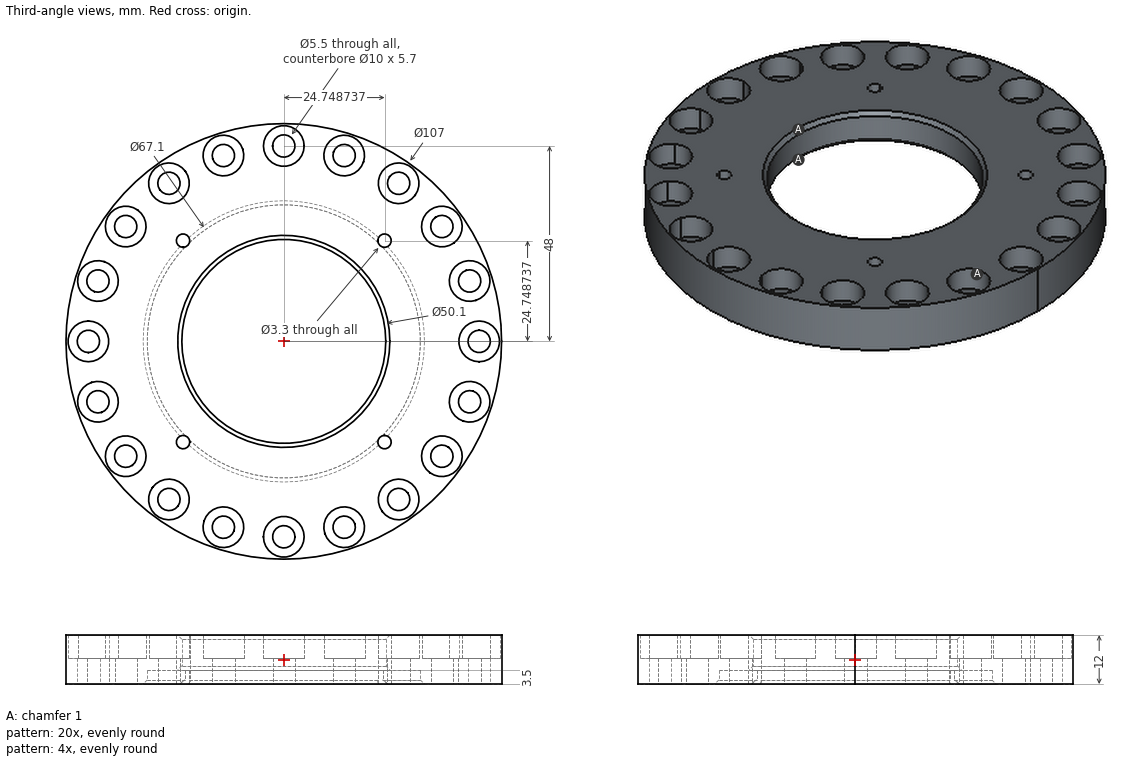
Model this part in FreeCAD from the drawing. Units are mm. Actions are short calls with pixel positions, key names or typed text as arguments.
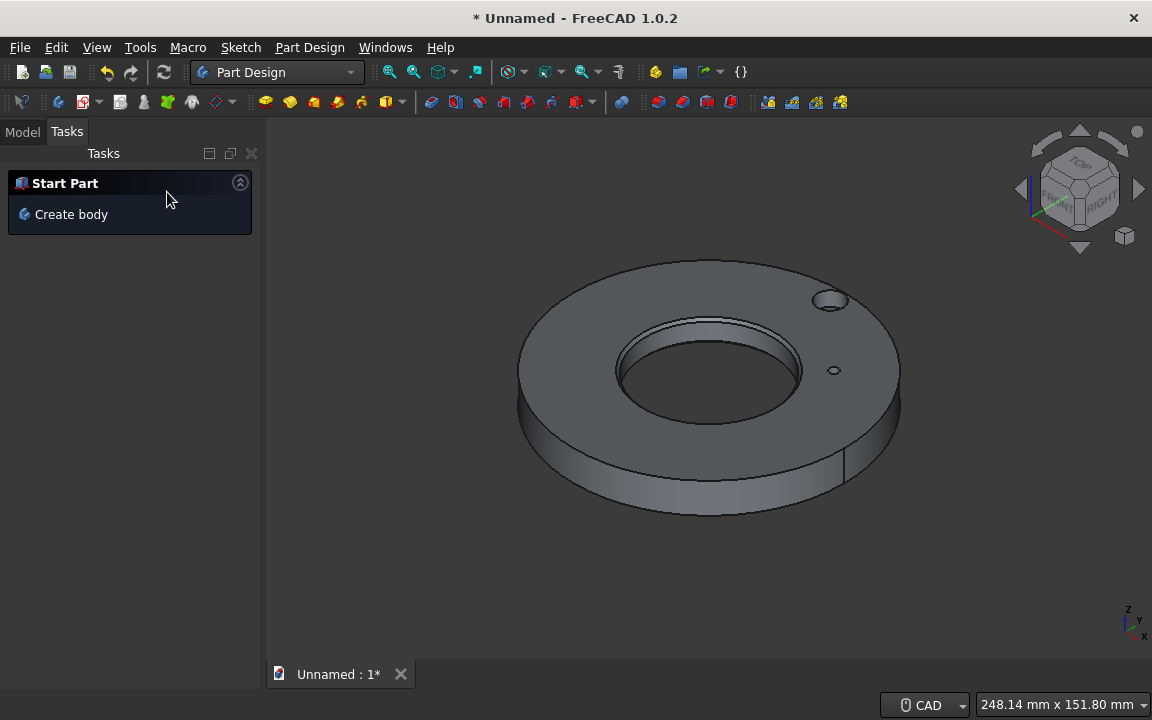
click(23, 131)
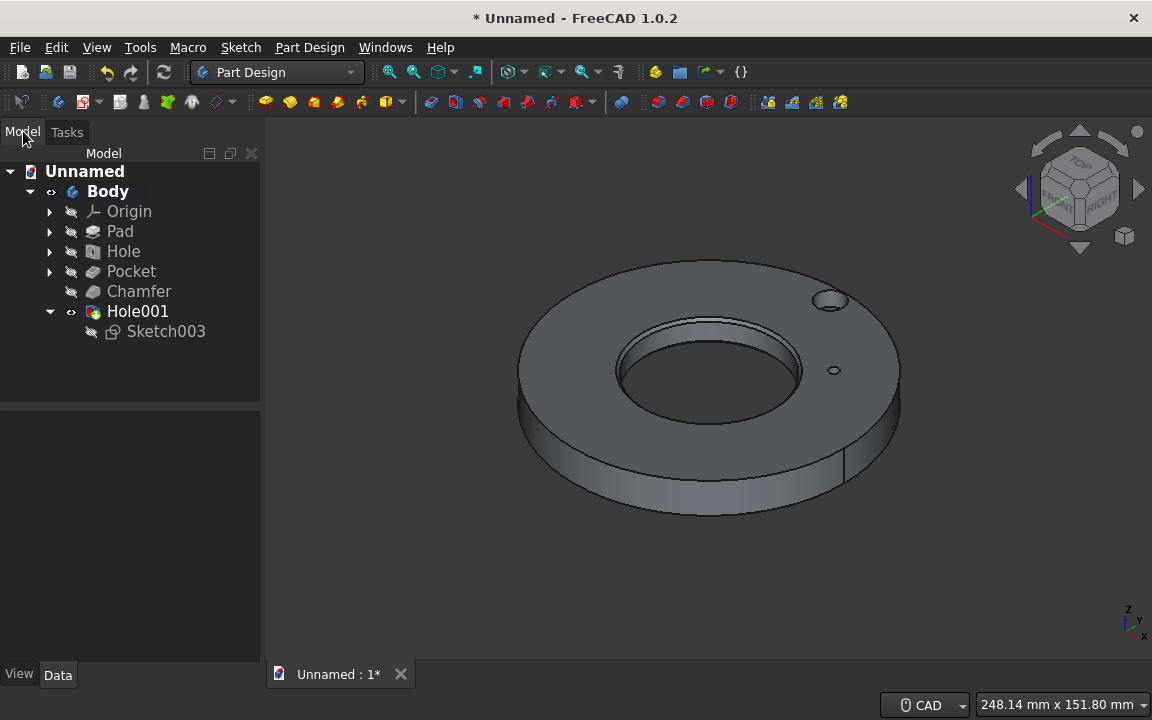
click(116, 252)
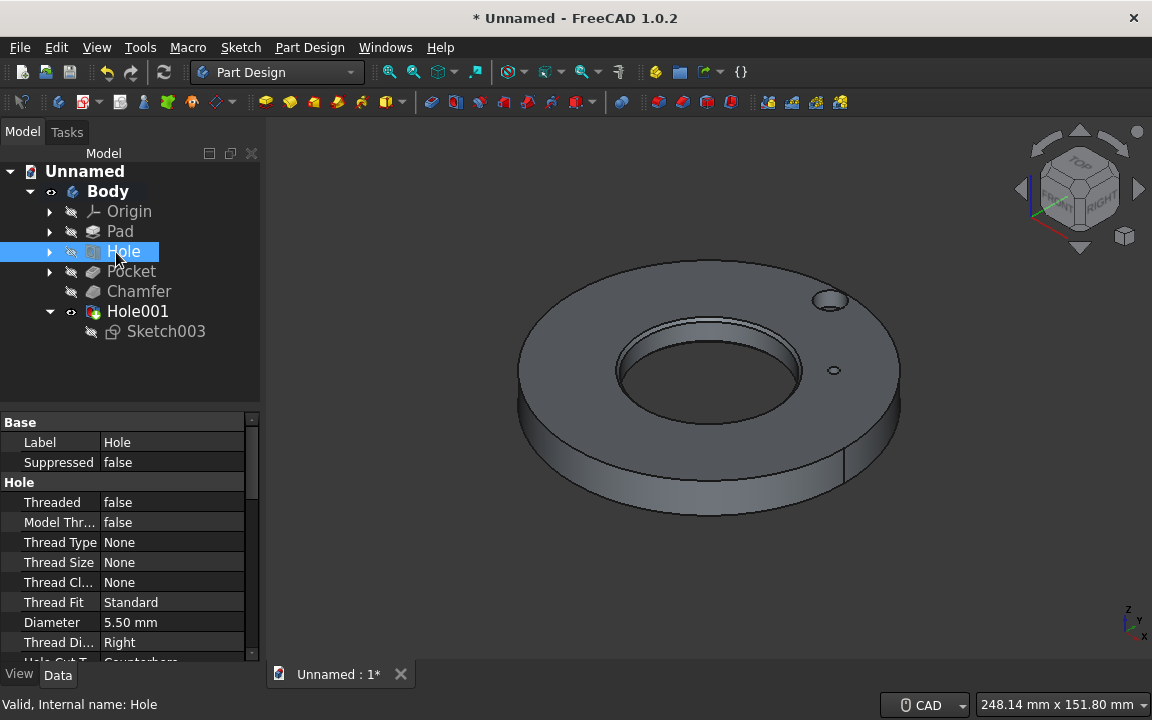
click(816, 102)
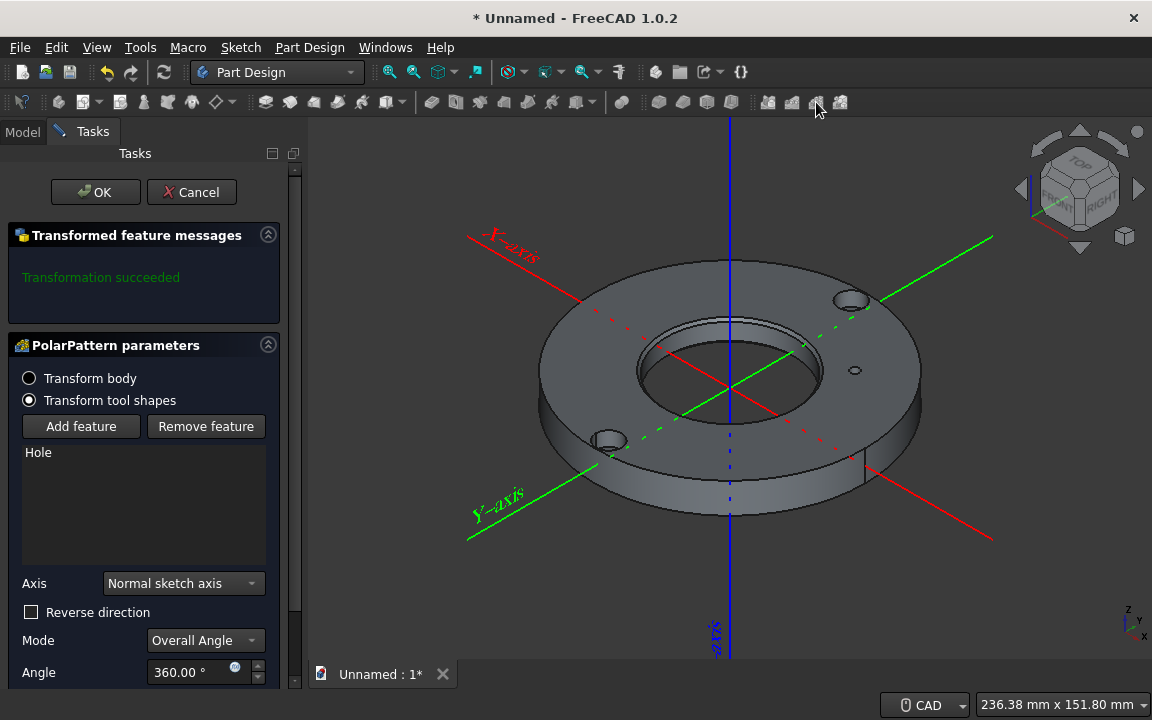
click(184, 584)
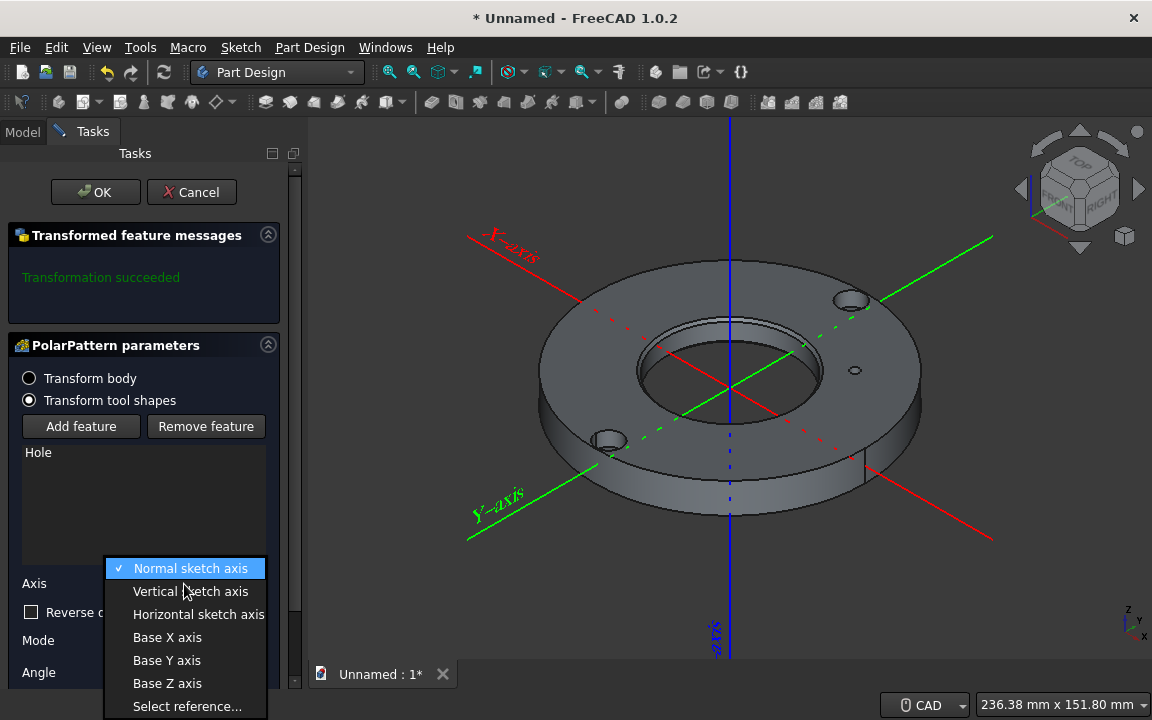
click(184, 684)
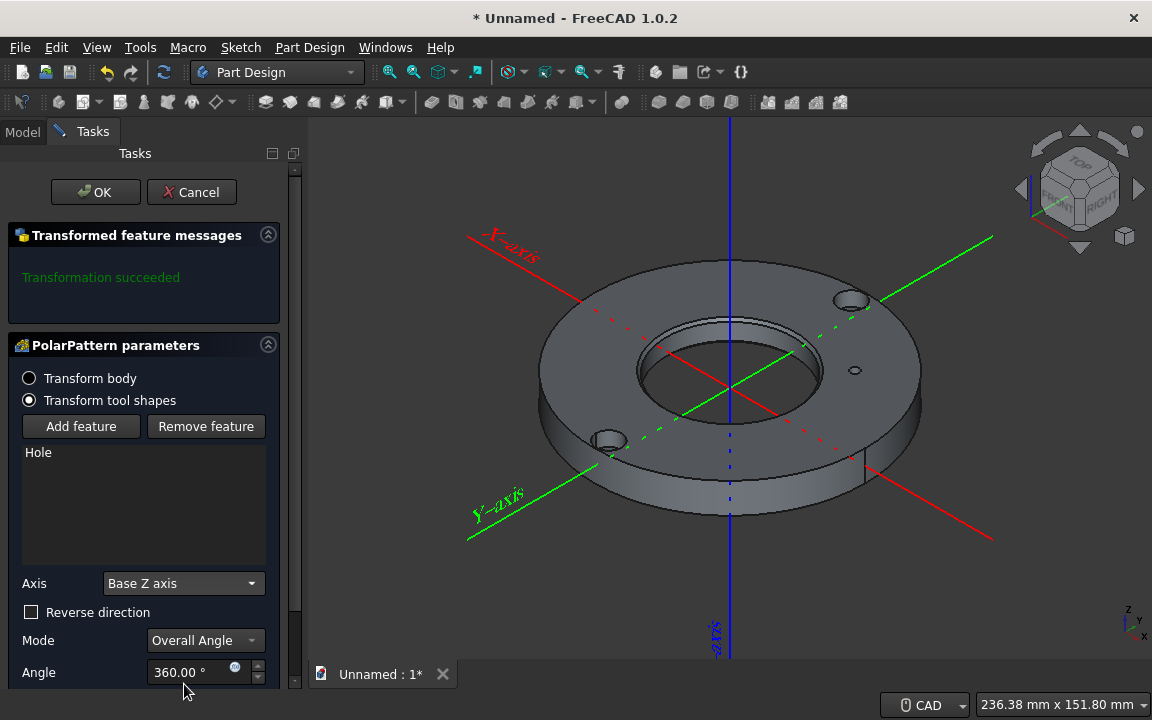
scroll(295, 426, down, 2)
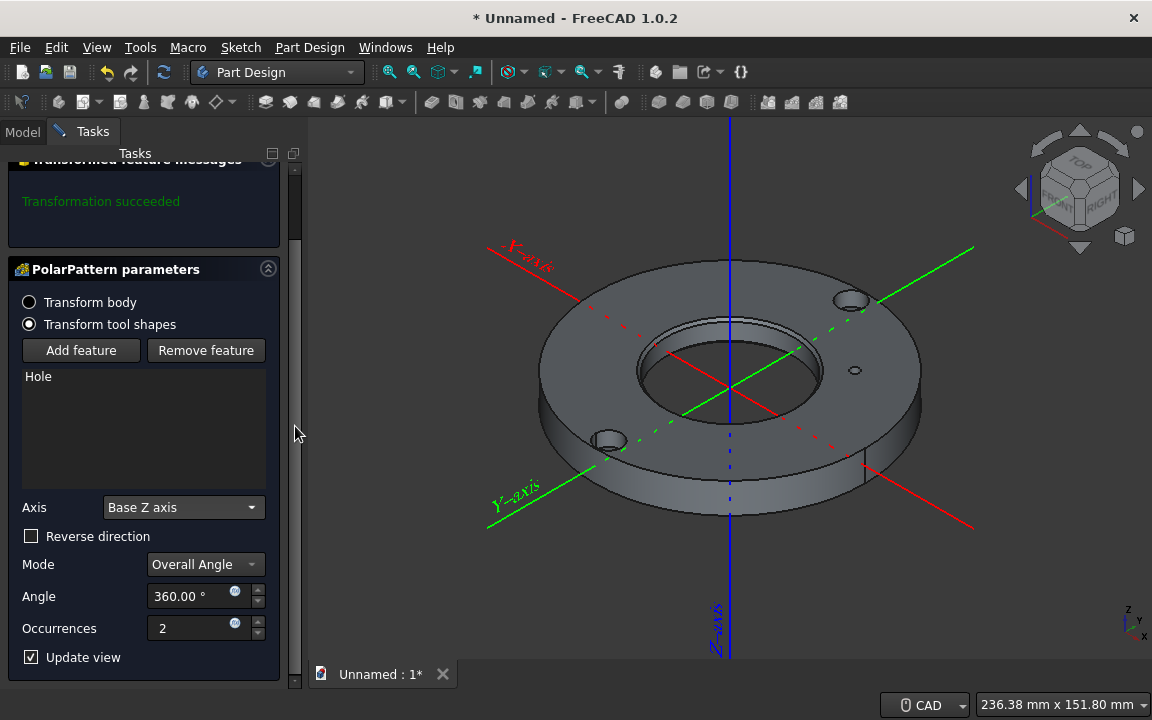
triple_click(198, 628)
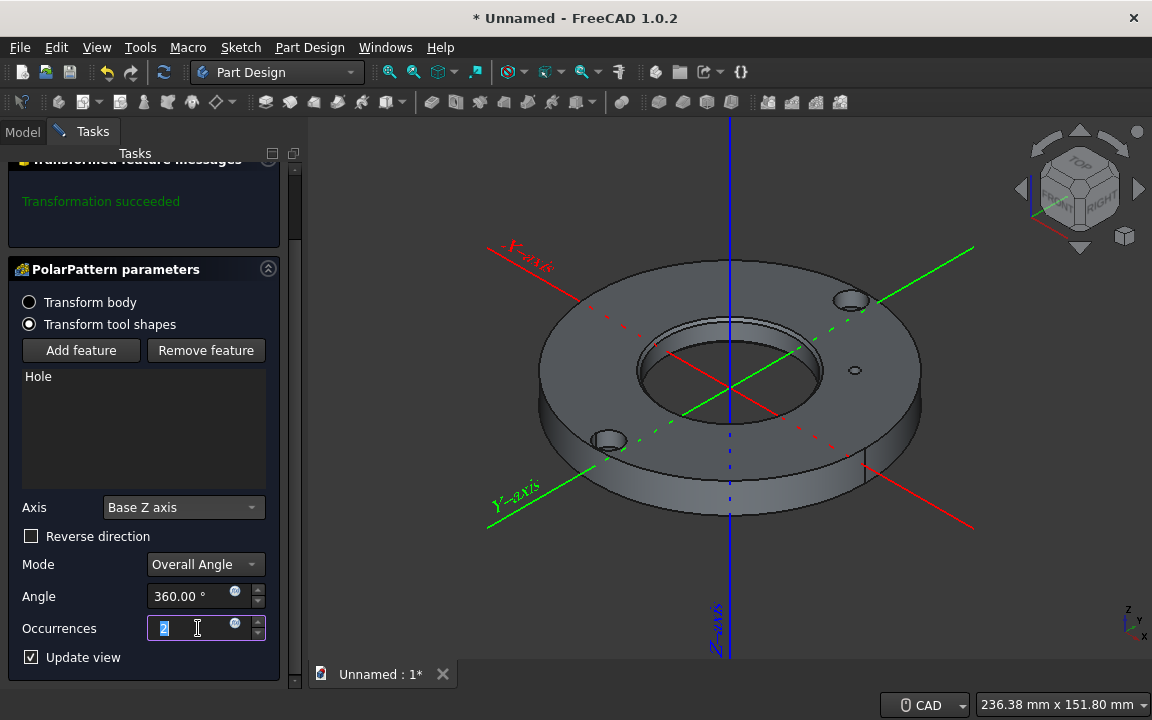
text(20)
key(Tab)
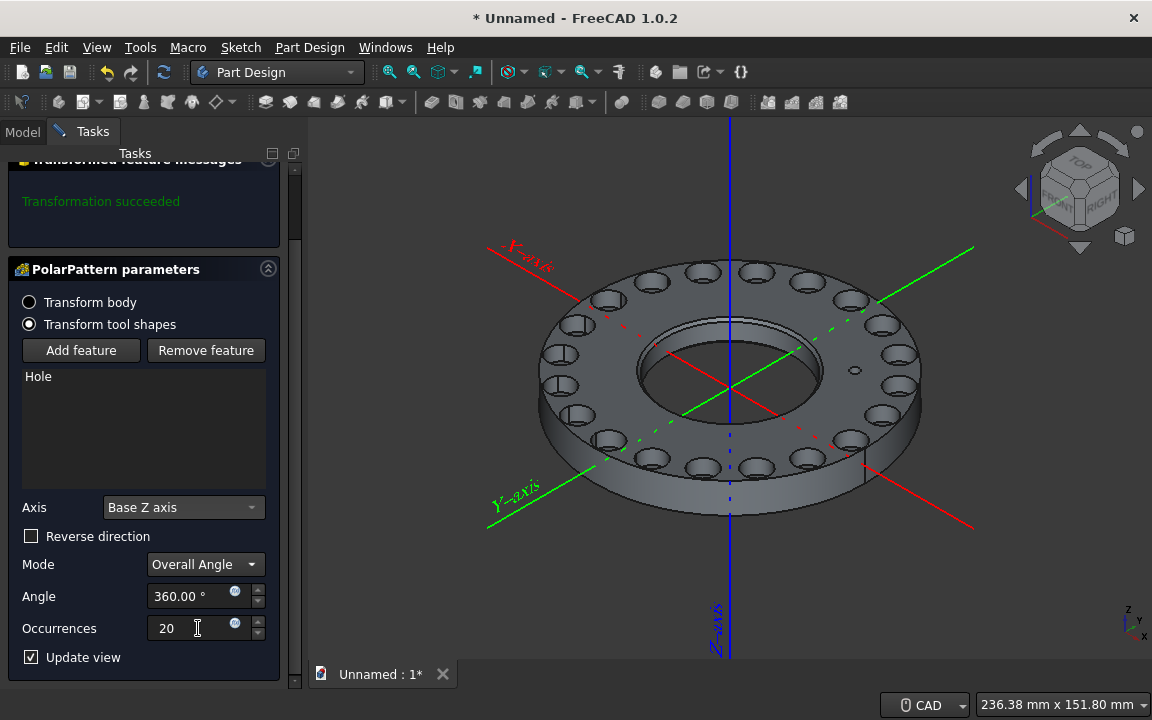
scroll(295, 426, up, 3)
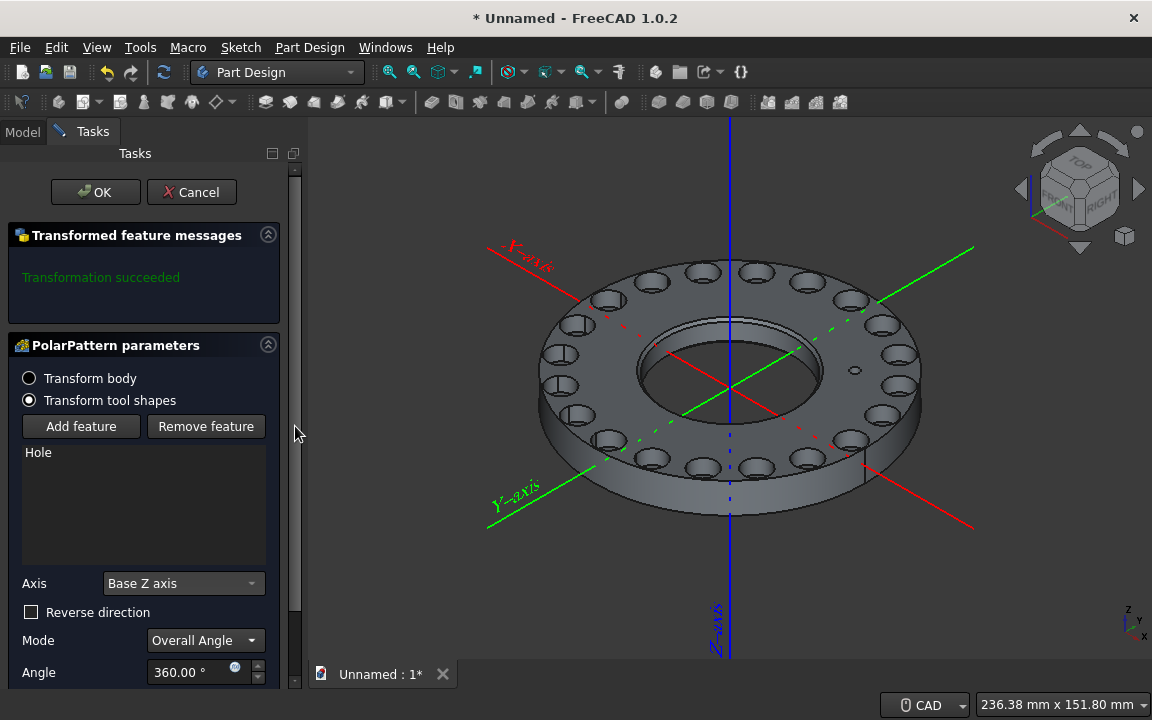
click(96, 192)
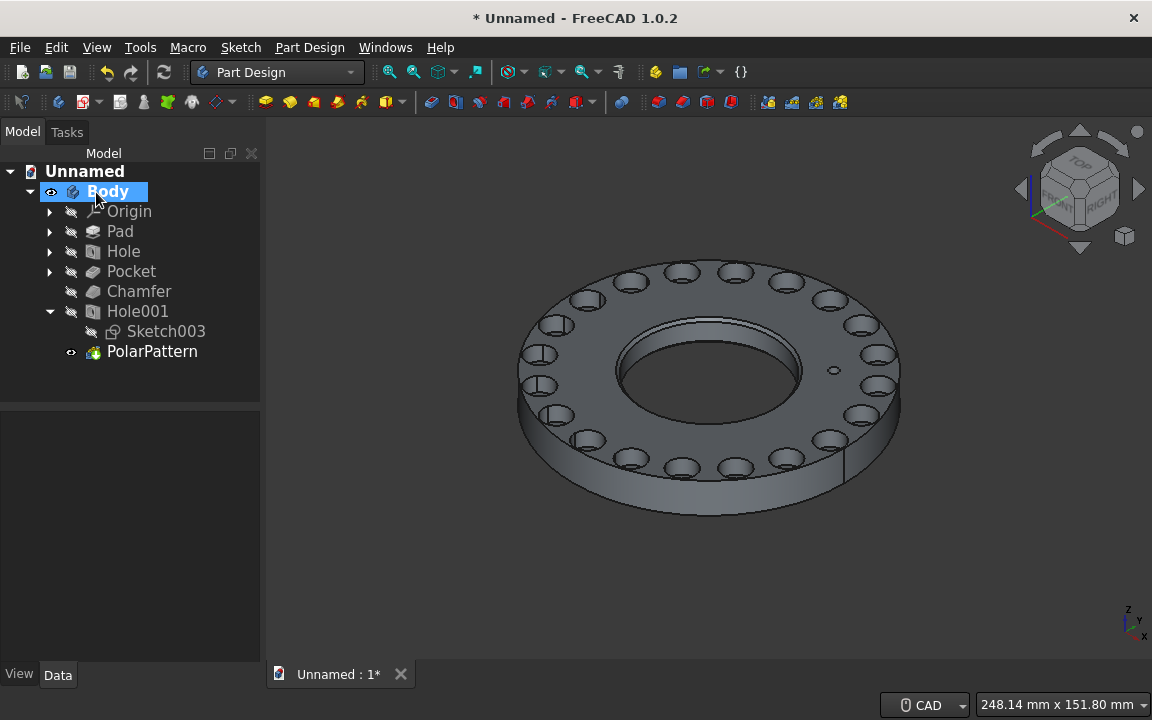
click(116, 312)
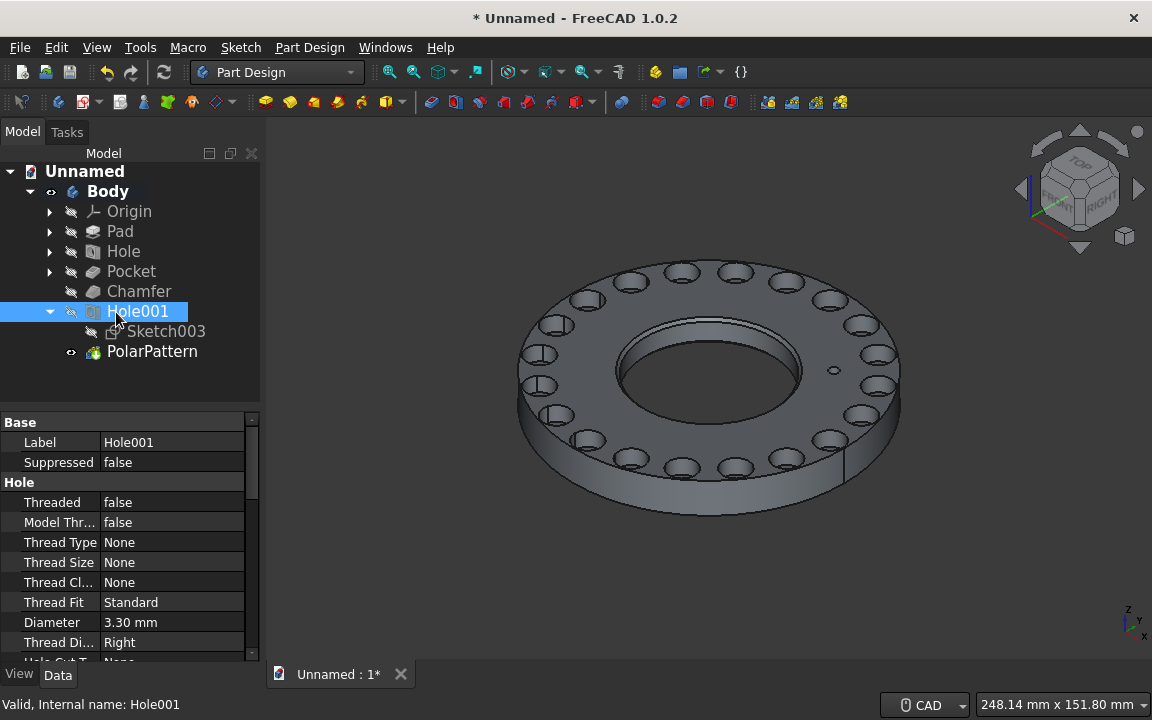
click(816, 102)